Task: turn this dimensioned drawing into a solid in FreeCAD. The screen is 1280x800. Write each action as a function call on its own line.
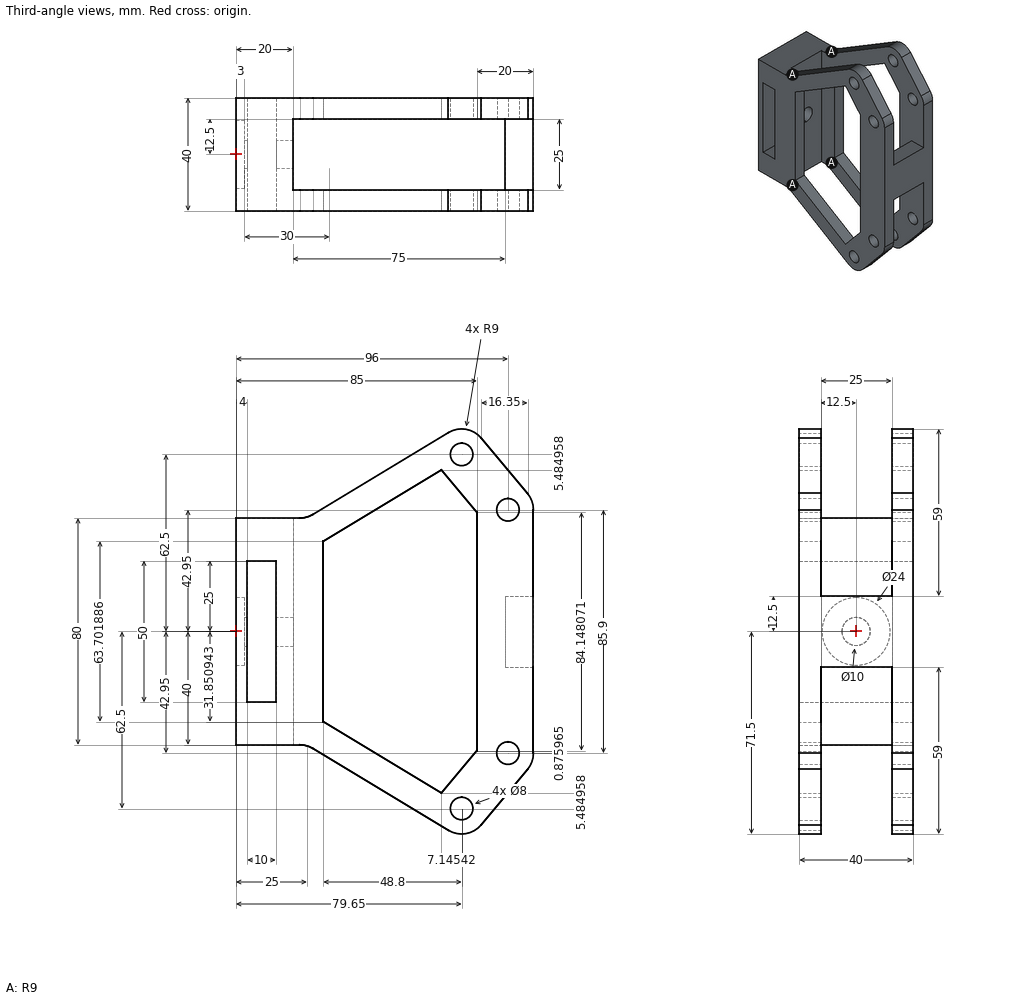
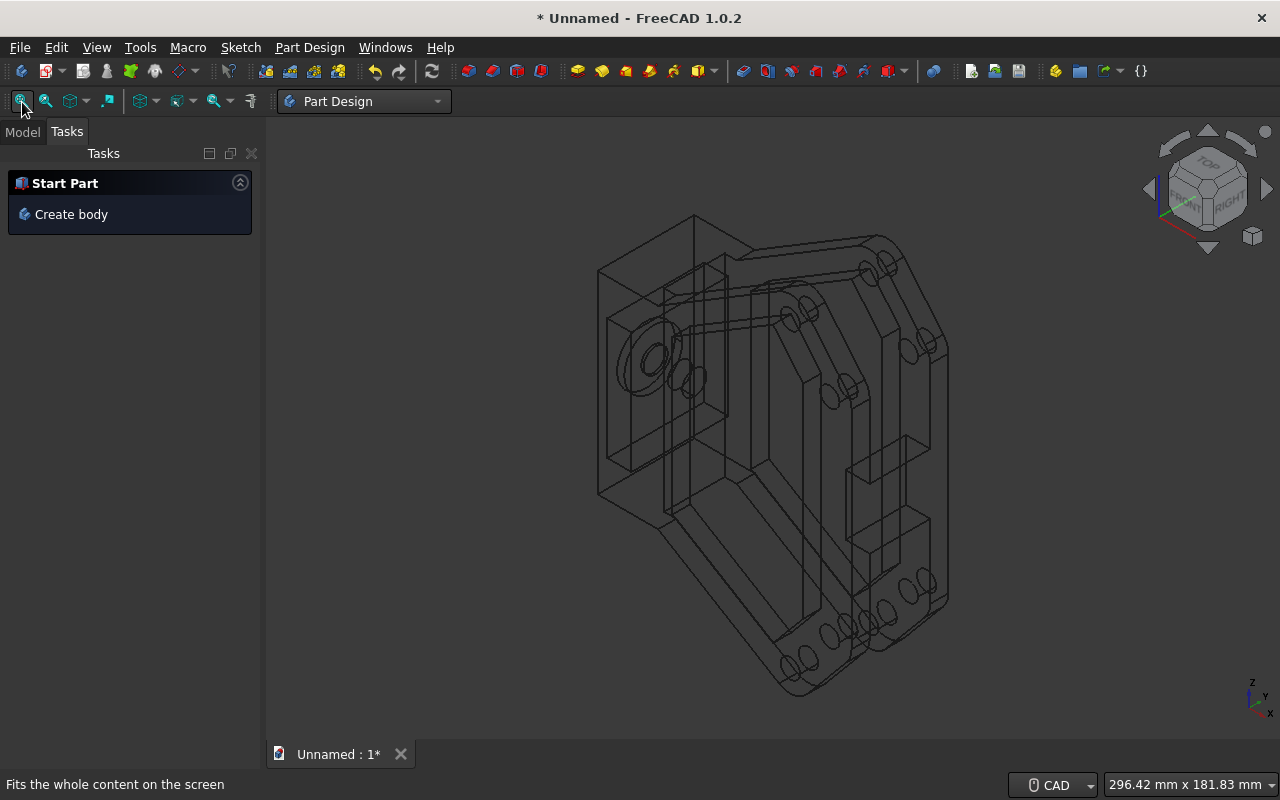
click(667, 523)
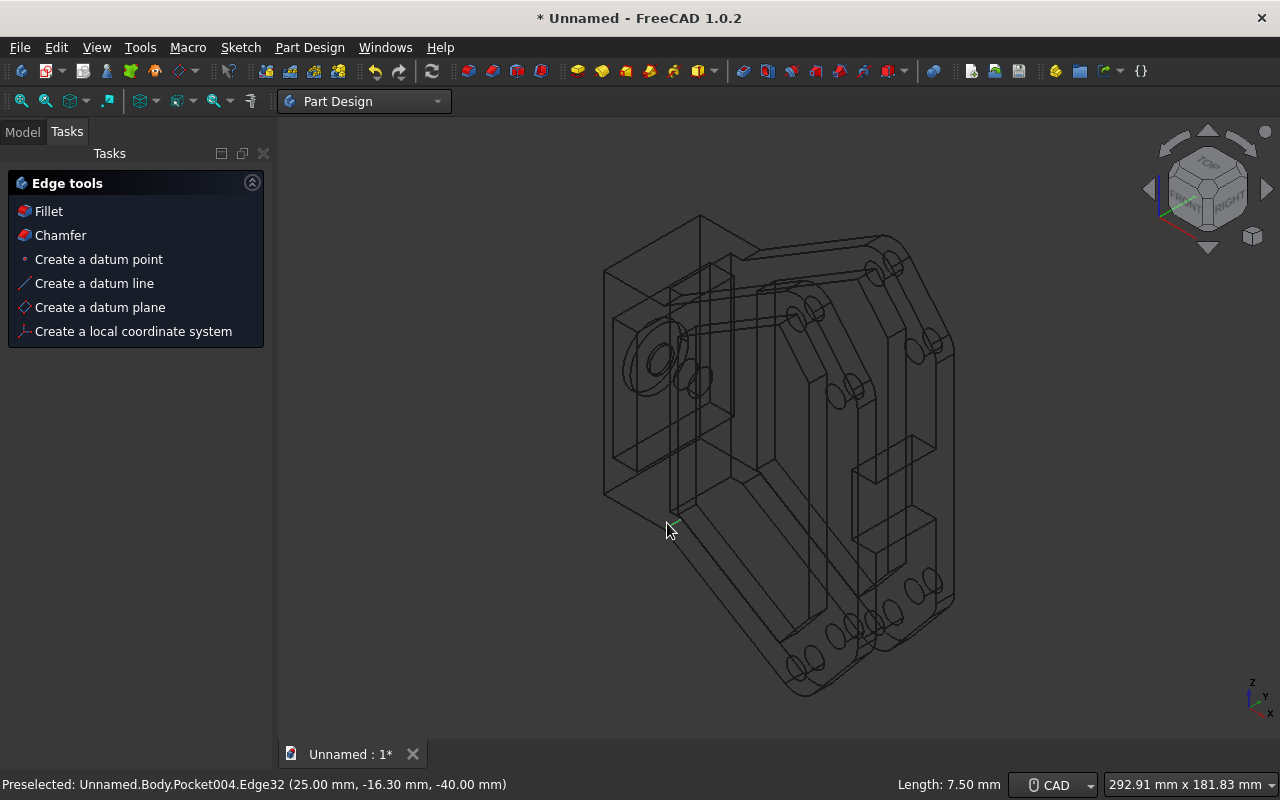
click(677, 297, ctrl)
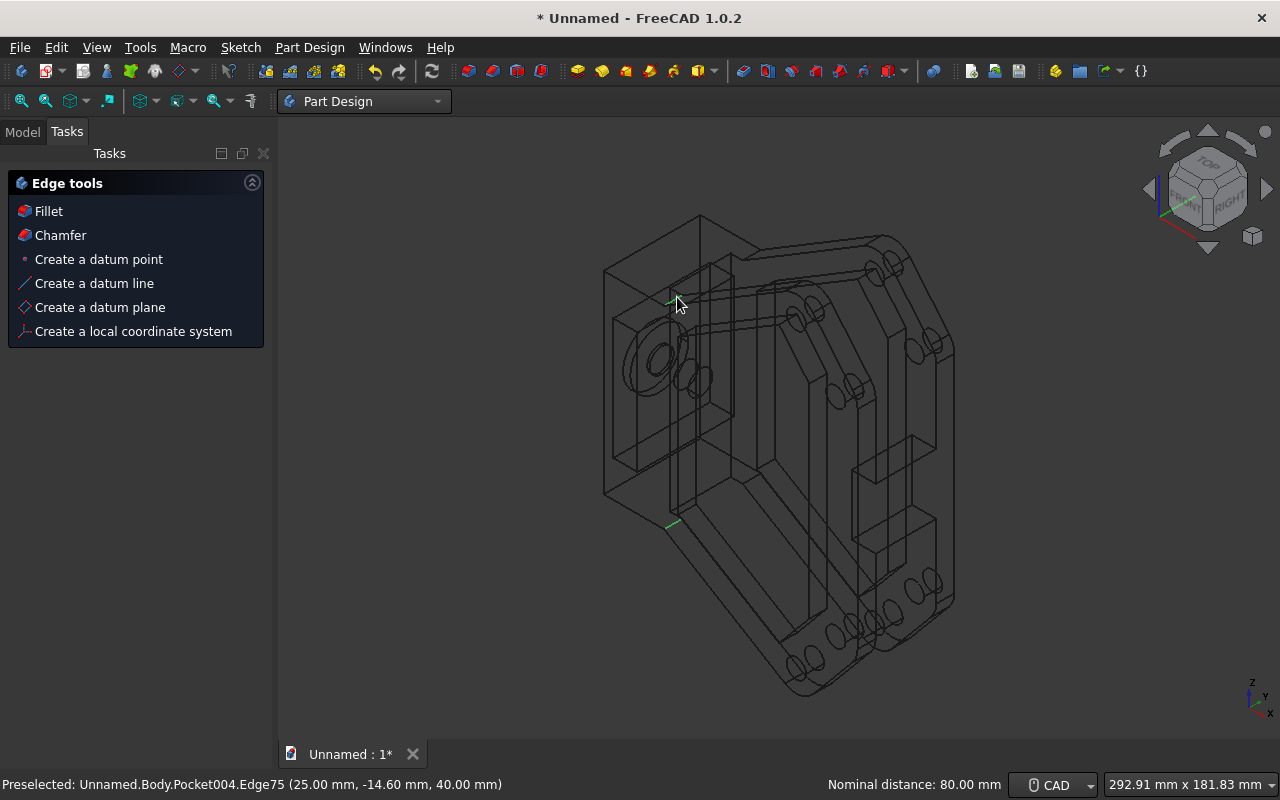
click(752, 478, ctrl)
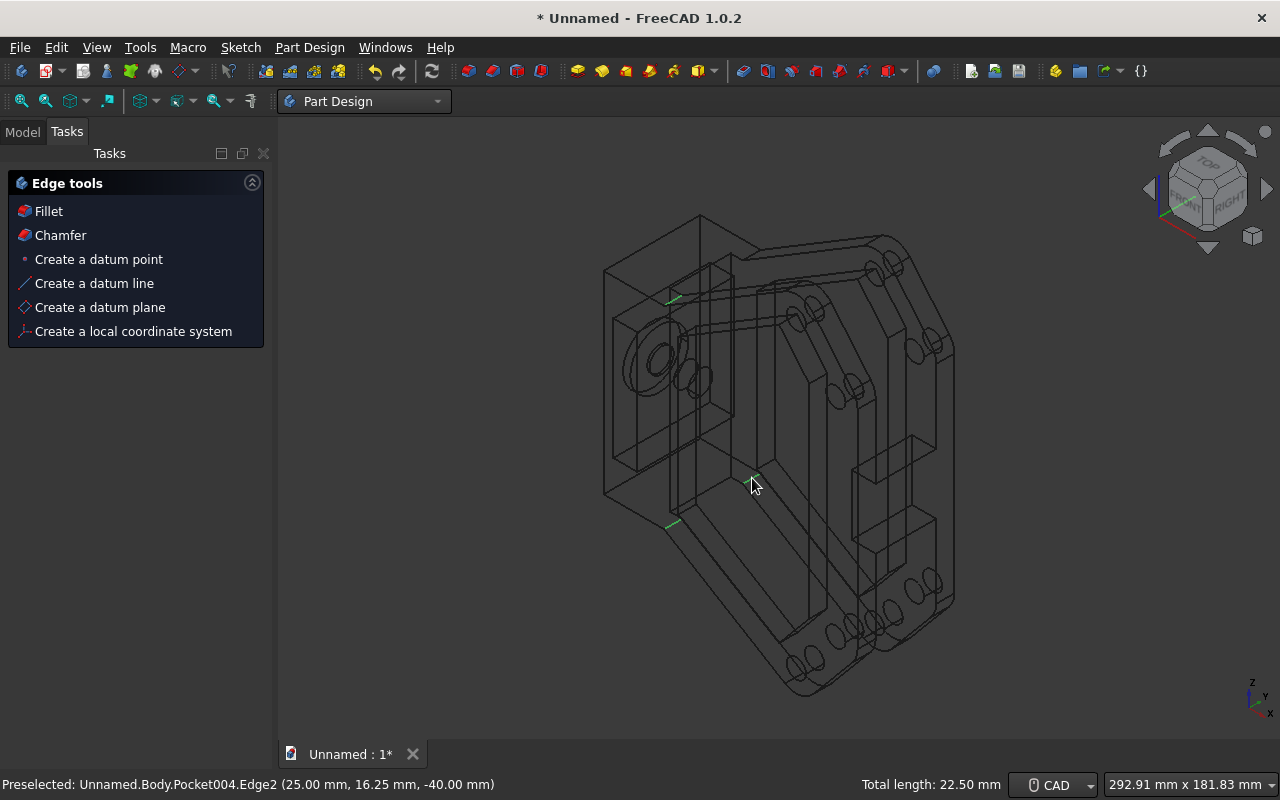
click(757, 251, ctrl)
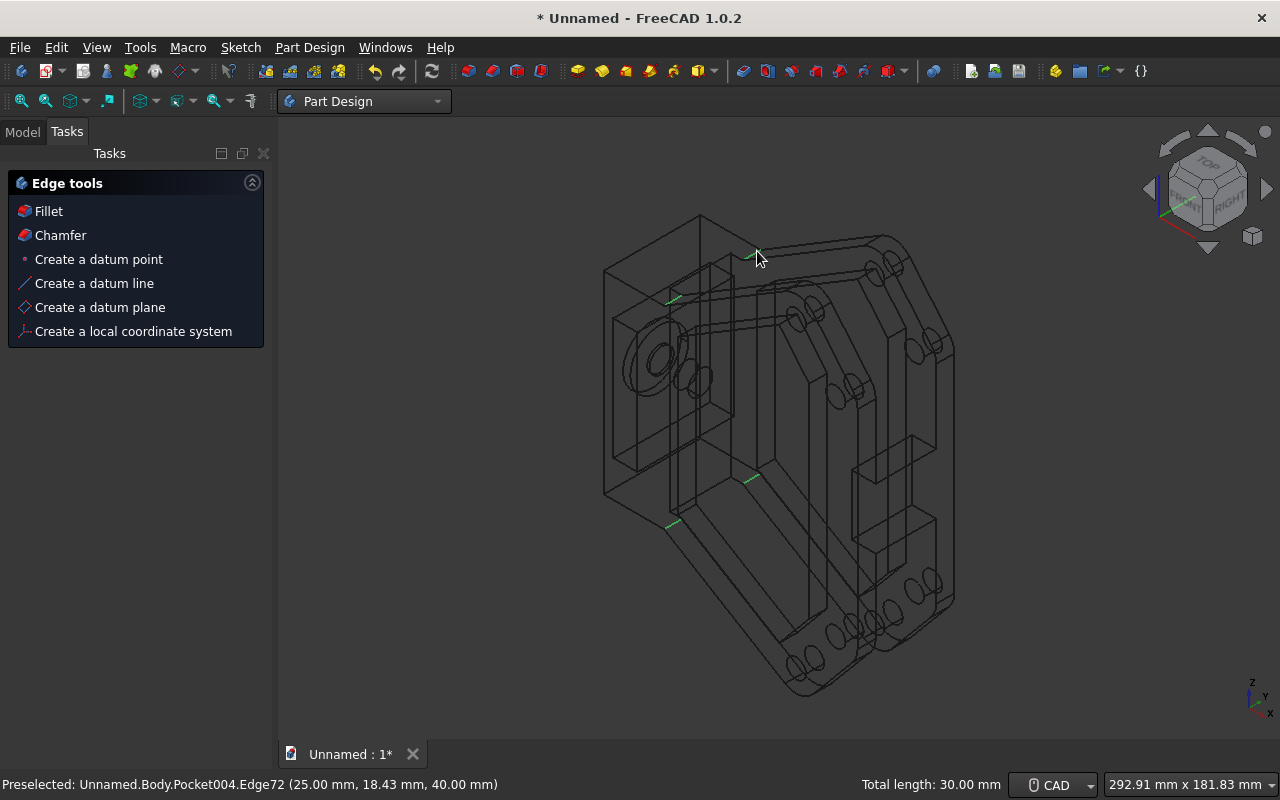
key(v)
key(1)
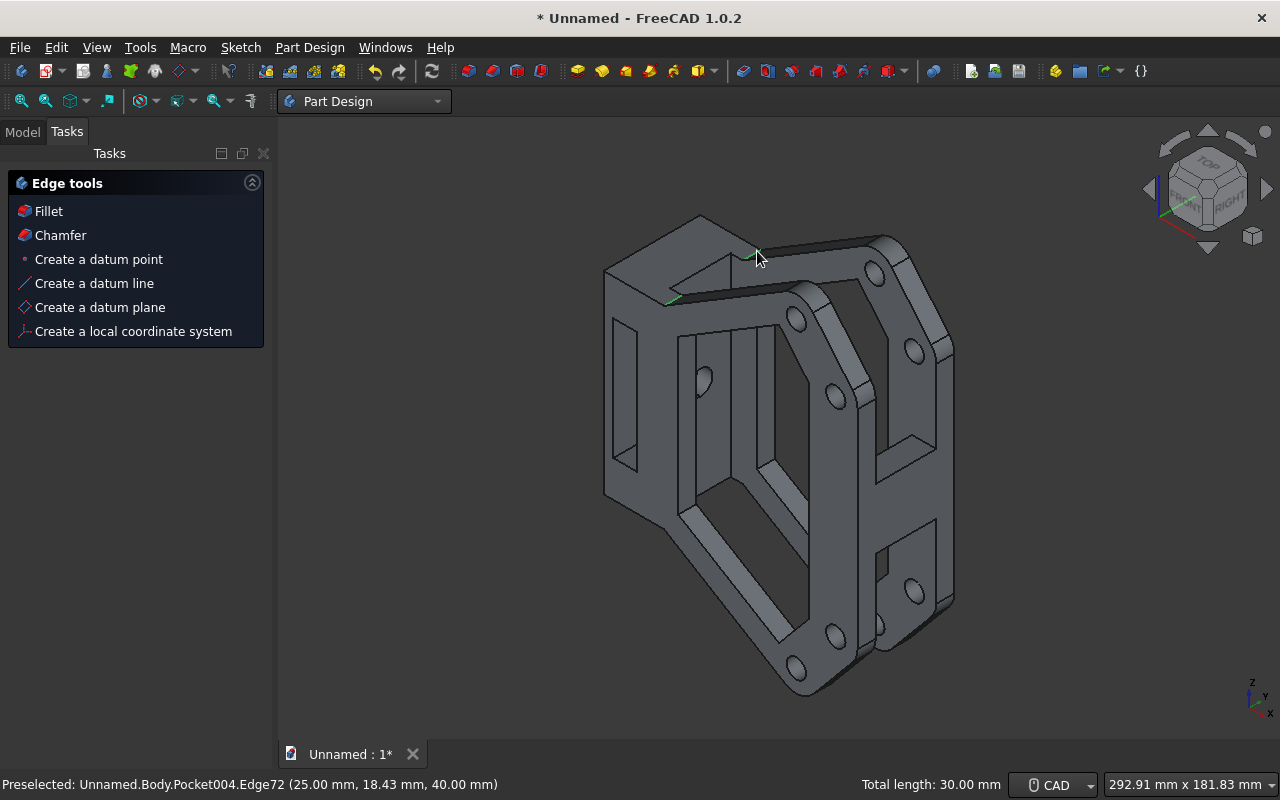
click(470, 72)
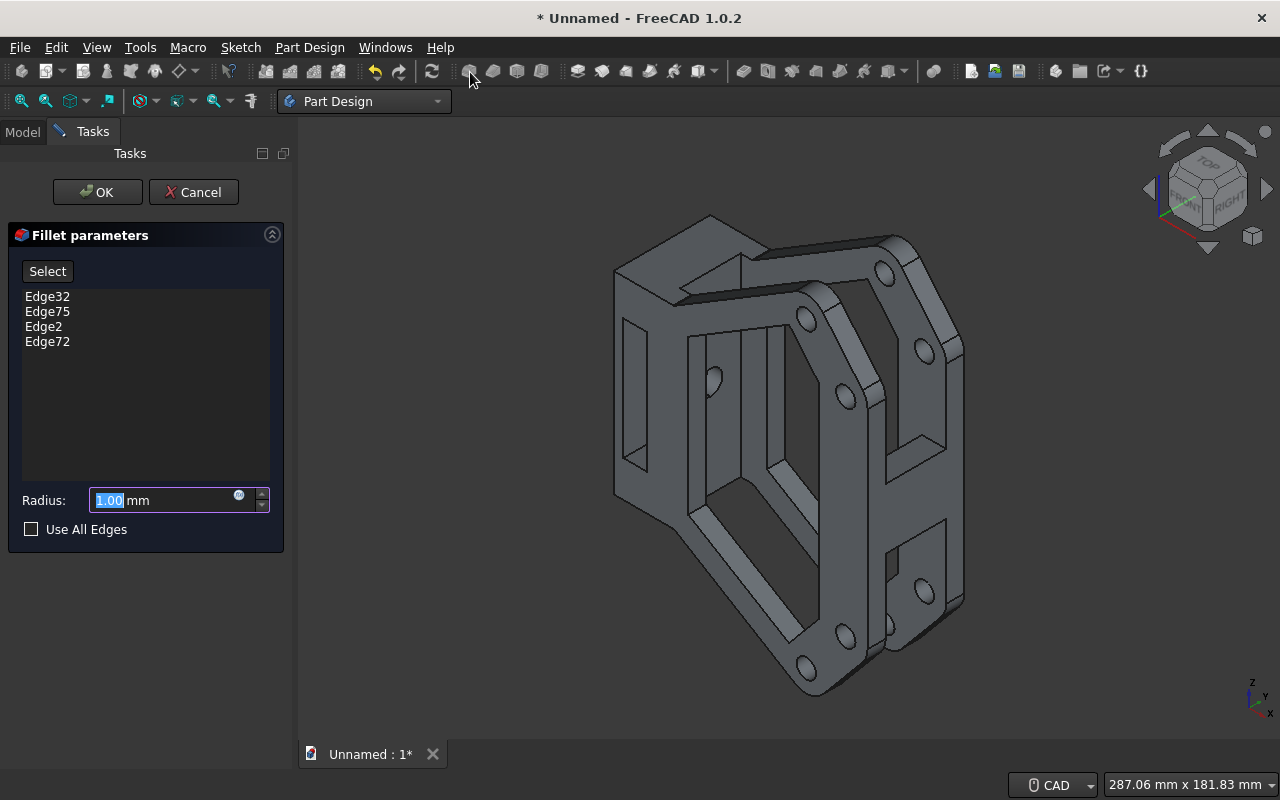
text(9)
key(Tab)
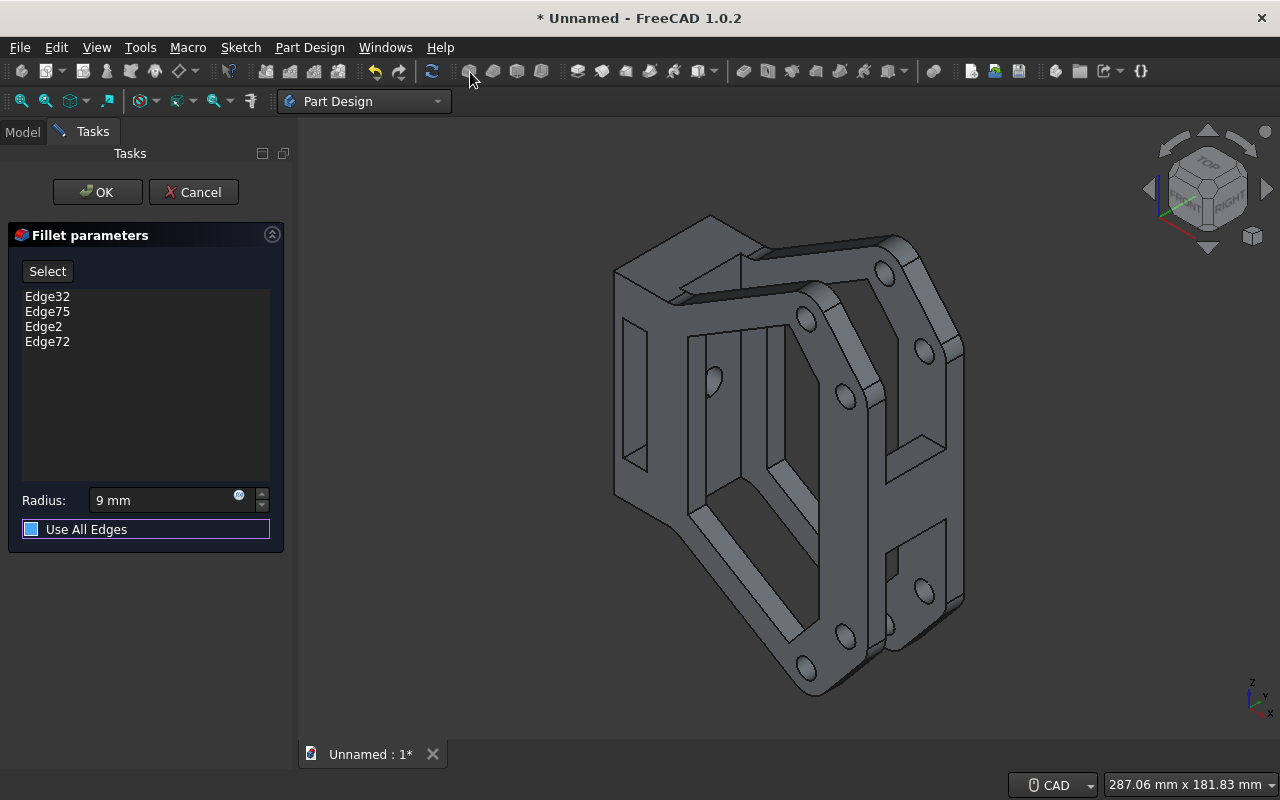
click(98, 192)